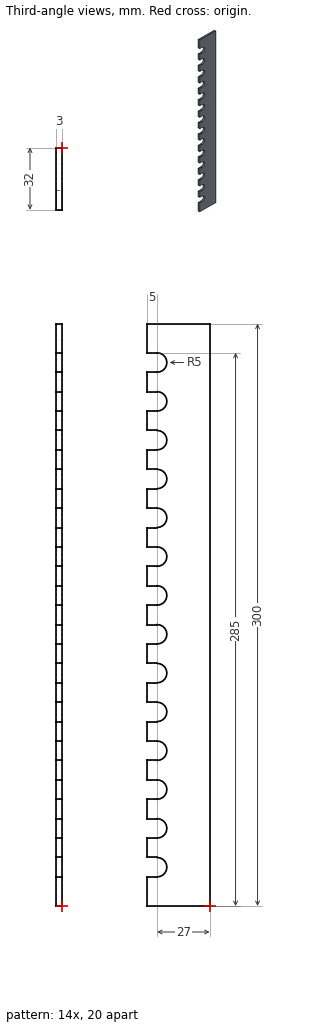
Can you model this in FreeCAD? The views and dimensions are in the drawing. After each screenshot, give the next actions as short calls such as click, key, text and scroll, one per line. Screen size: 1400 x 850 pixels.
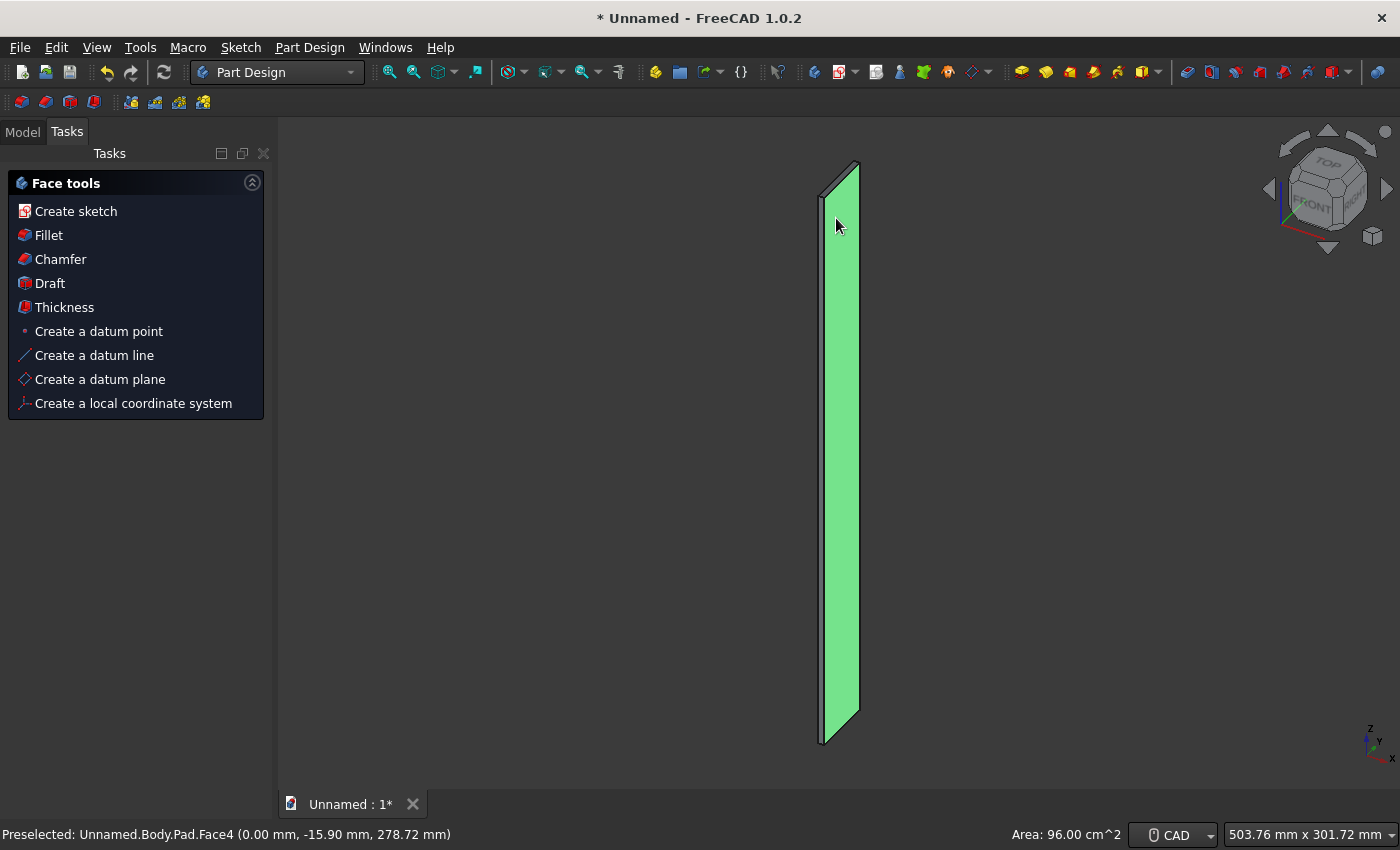
click(840, 72)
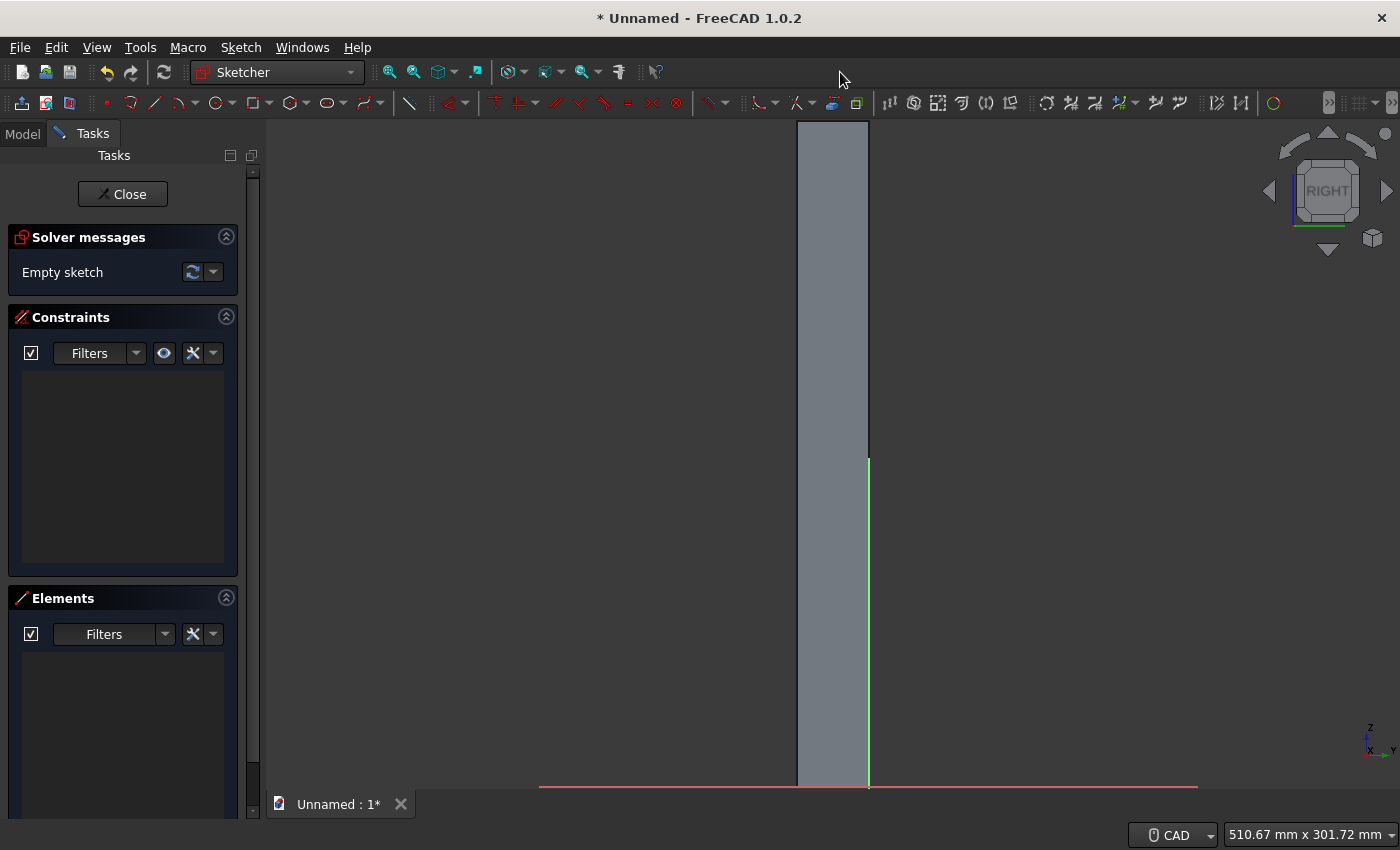
scroll(811, 150, up, 15)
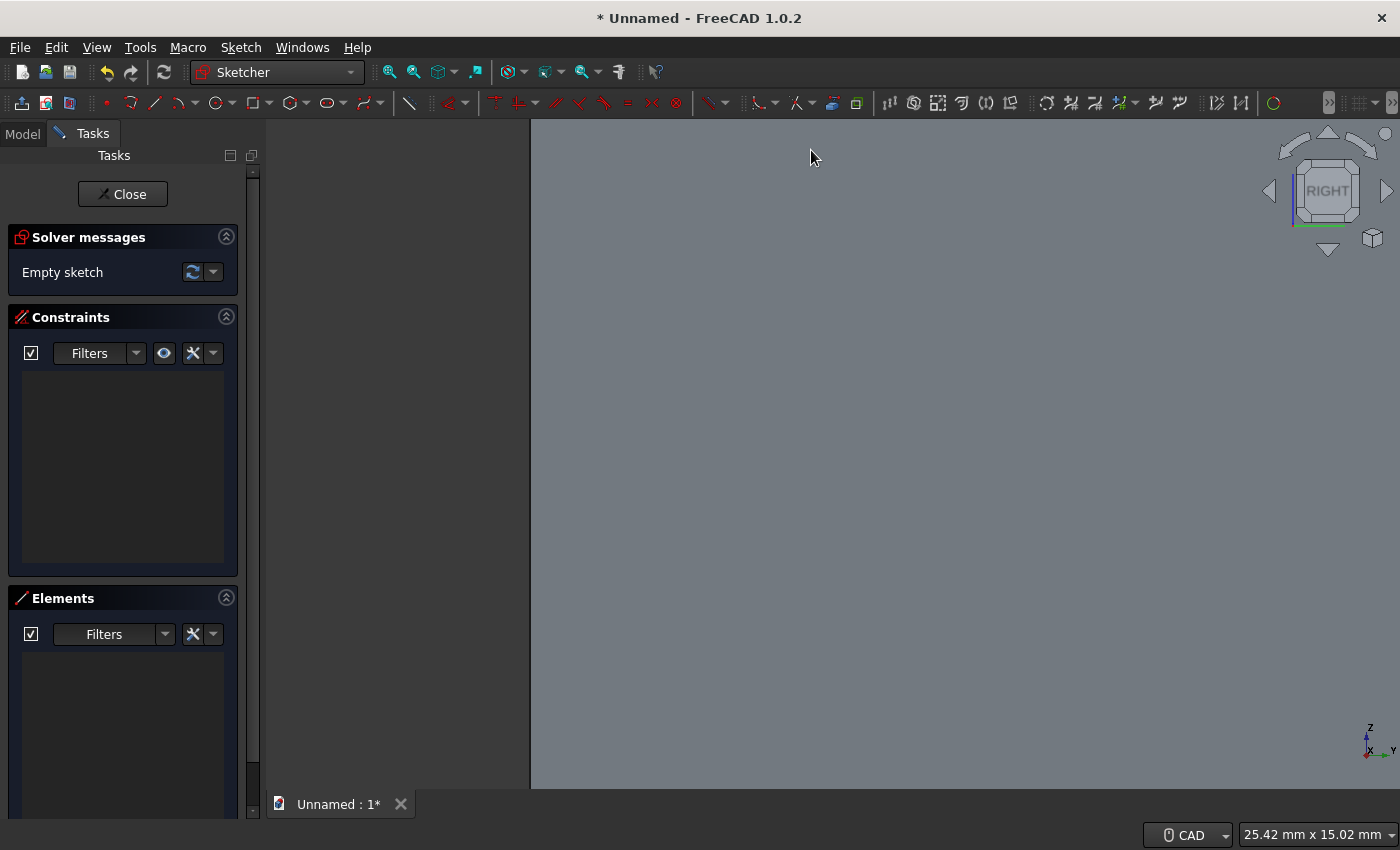
key(g)
key(m)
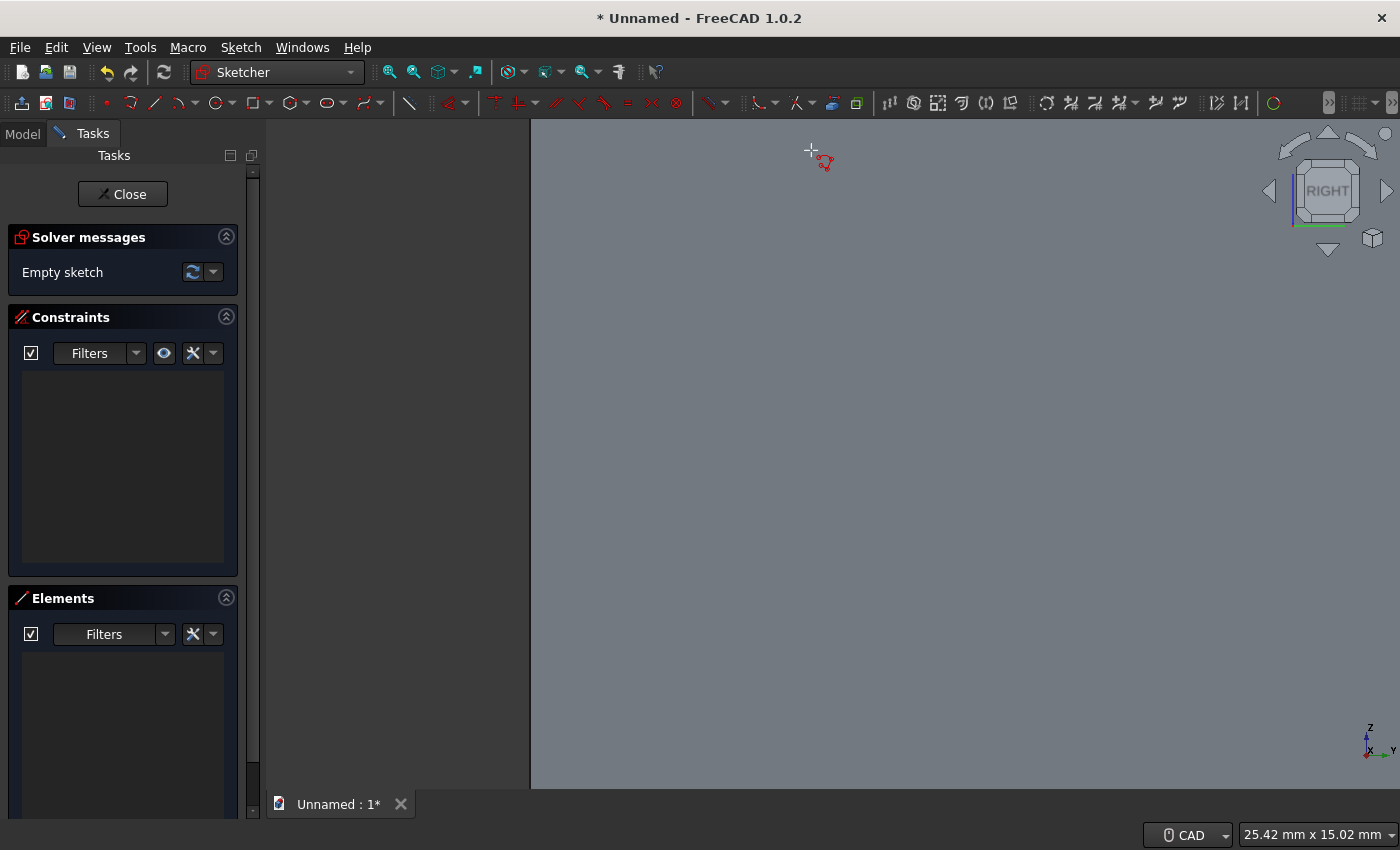
click(753, 234)
click(530, 234)
click(530, 680)
click(753, 680)
right_click(753, 680)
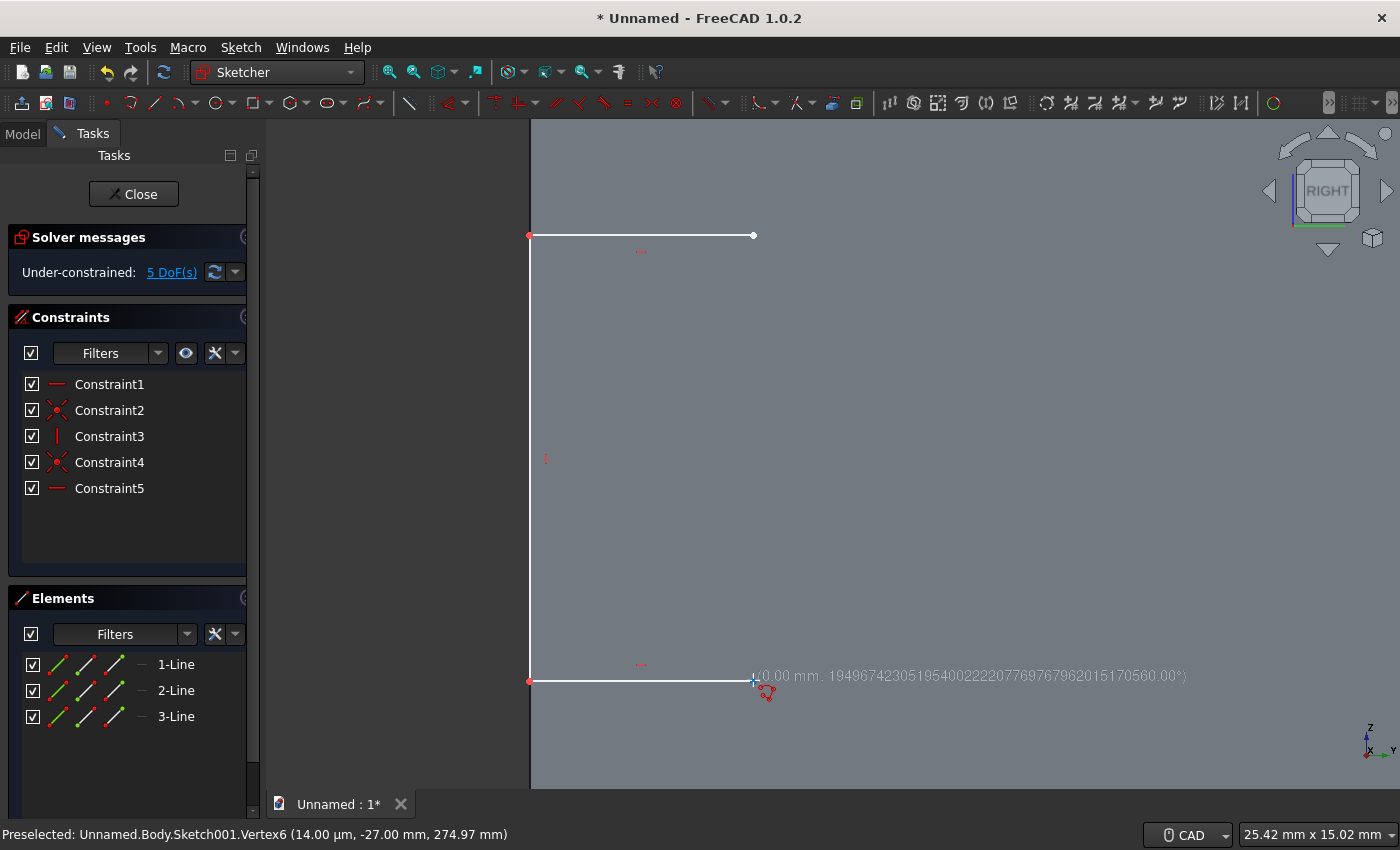
key(g)
key(3)
key(a)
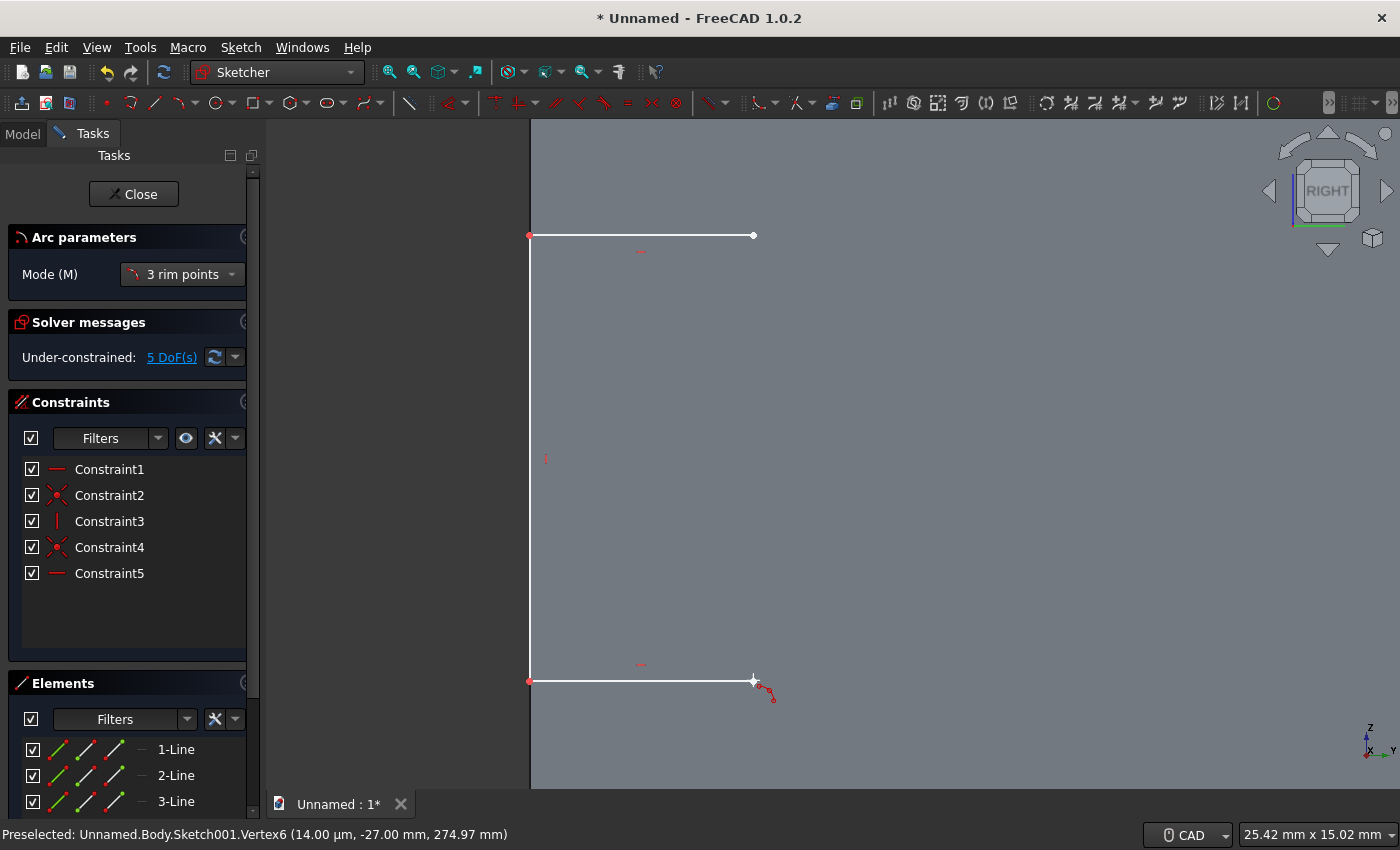
click(753, 681)
click(753, 235)
click(976, 457)
key(Escape)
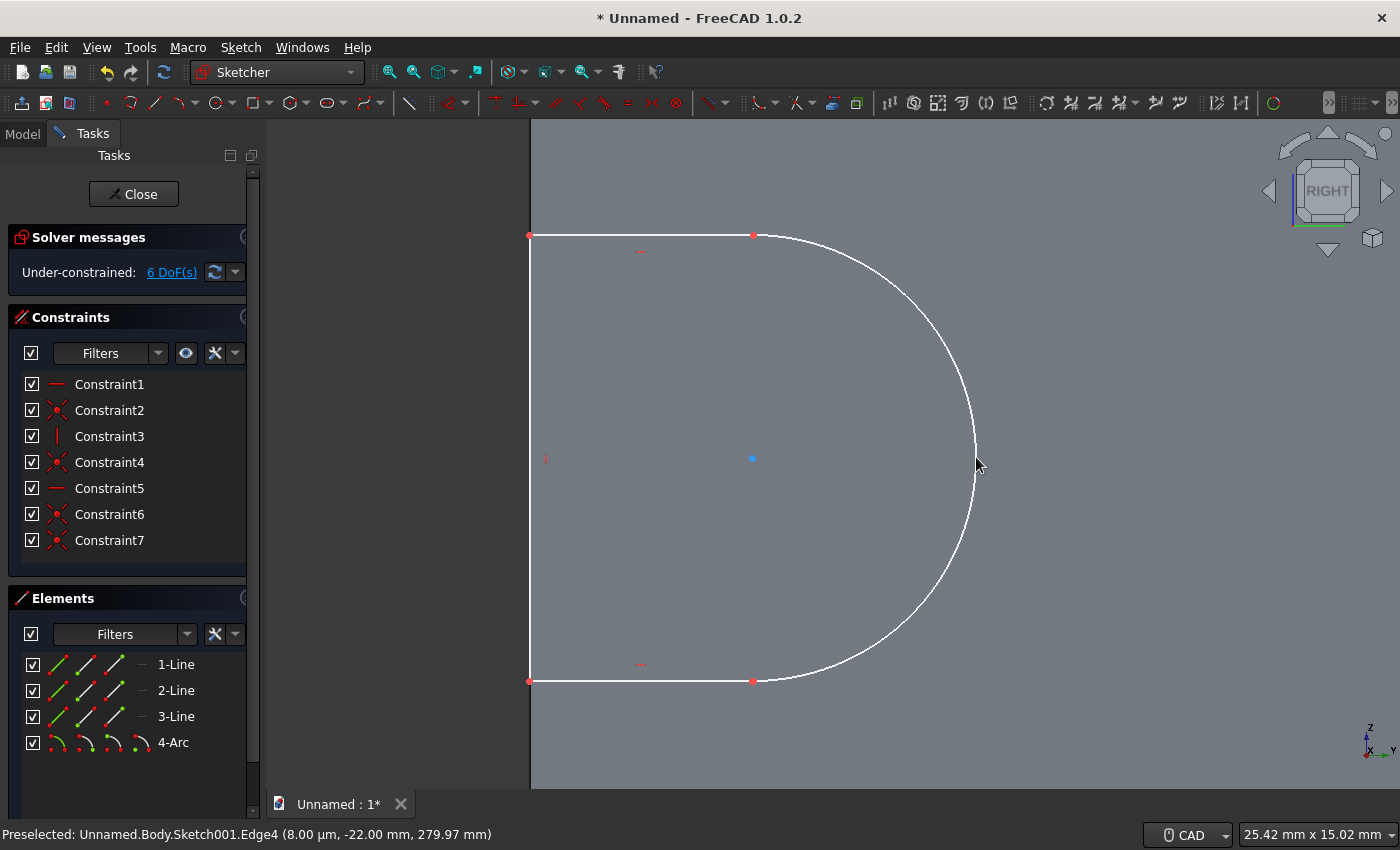
click(686, 235)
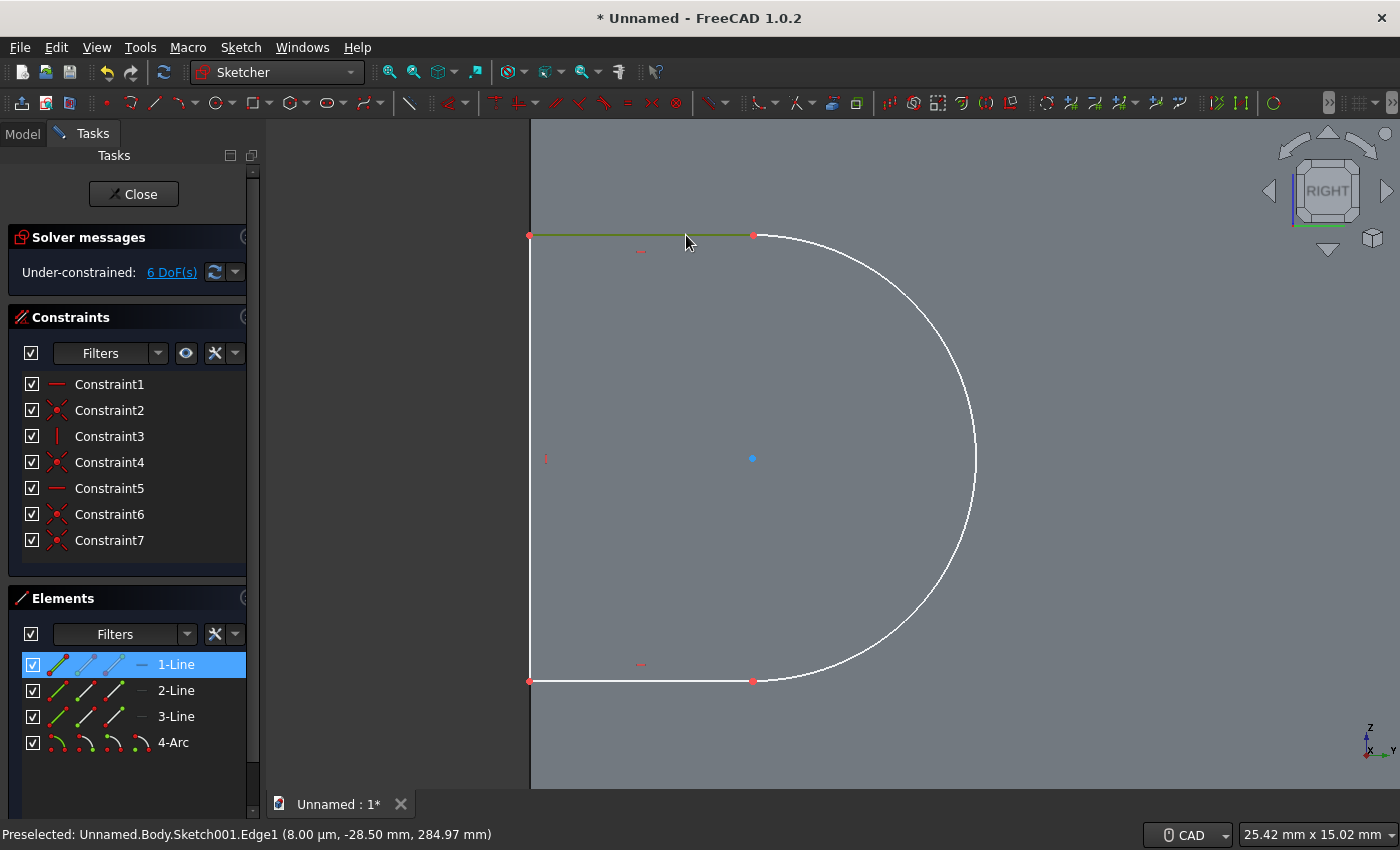
click(933, 589)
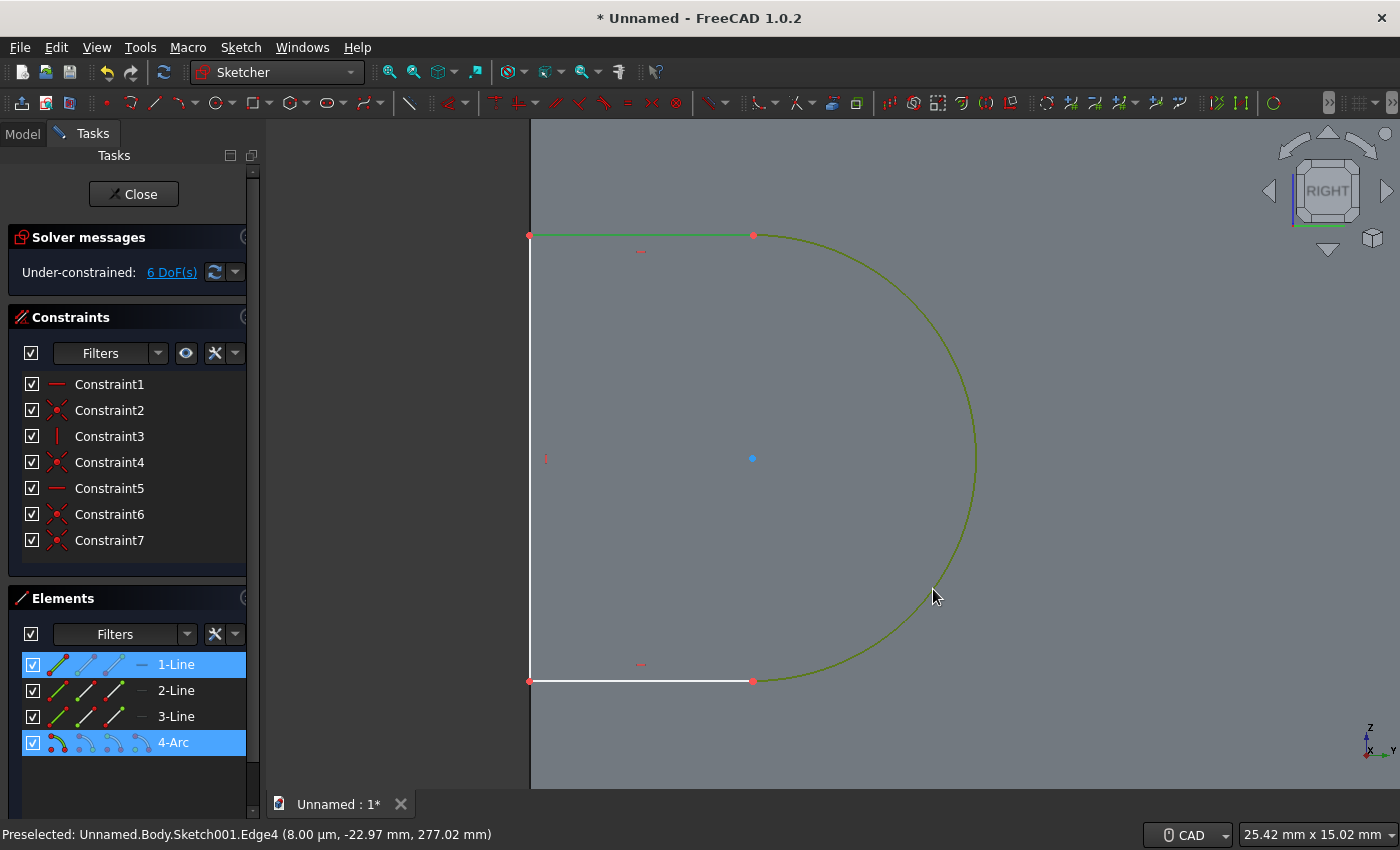
key(t)